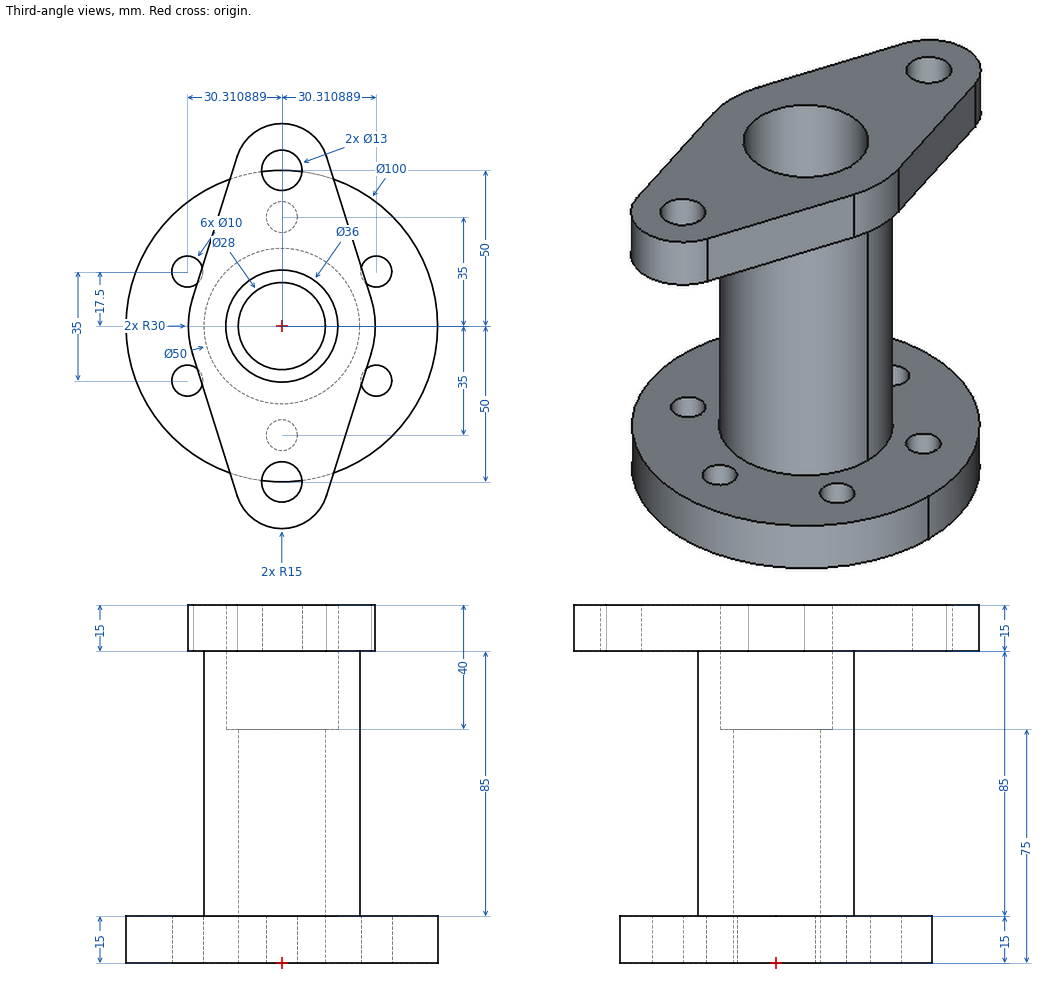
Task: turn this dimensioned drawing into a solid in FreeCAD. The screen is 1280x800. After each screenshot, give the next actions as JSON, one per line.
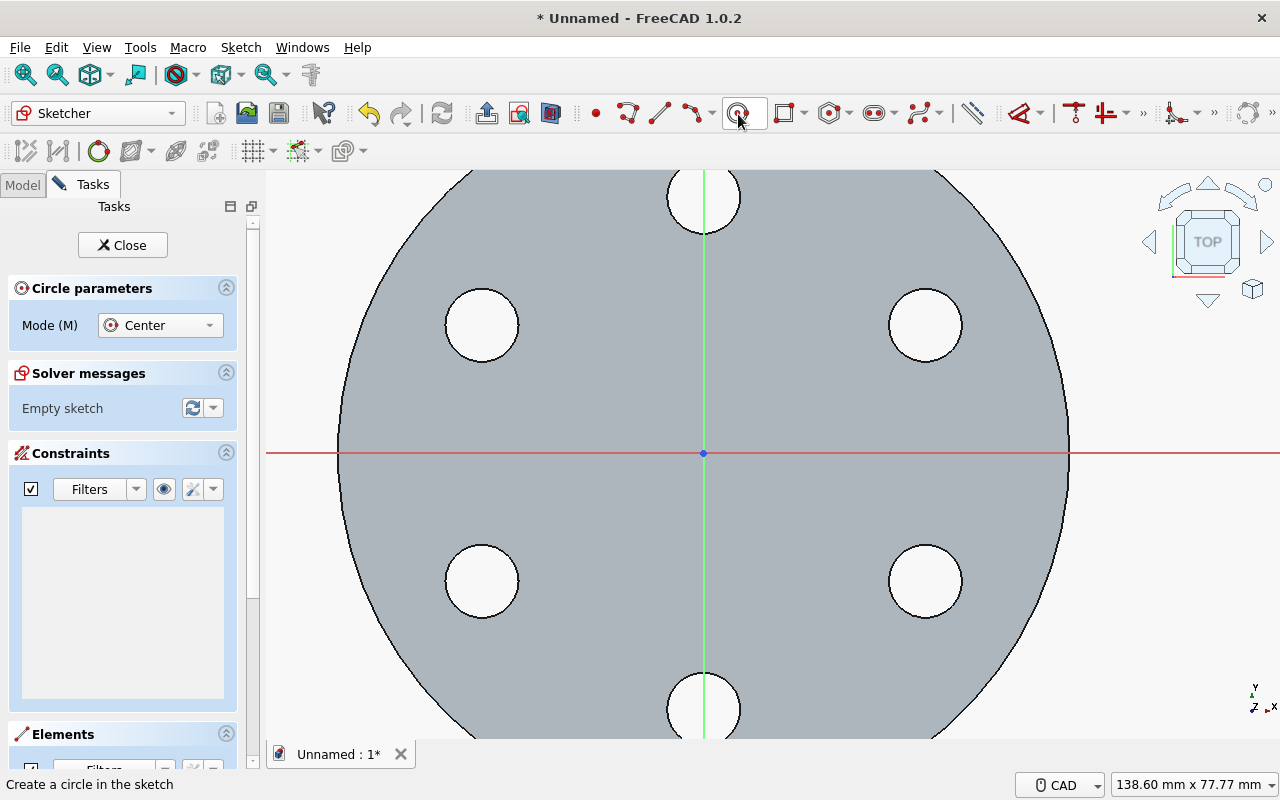
{"action": "left_click", "coordinate": [704, 453]}
{"action": "mouse_move", "coordinate": [833, 324]}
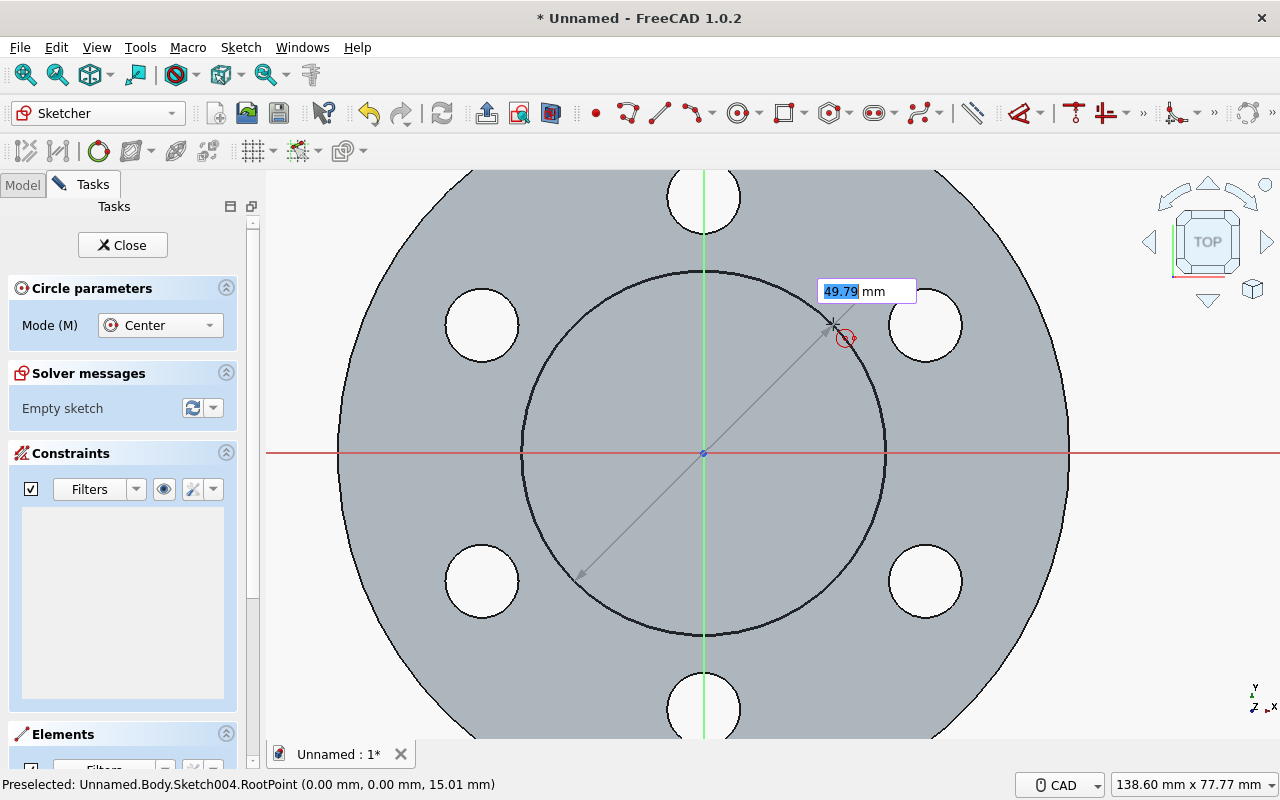
{"action": "type", "text": "50"}
{"action": "key", "text": "Return"}
{"action": "key", "text": "Escape"}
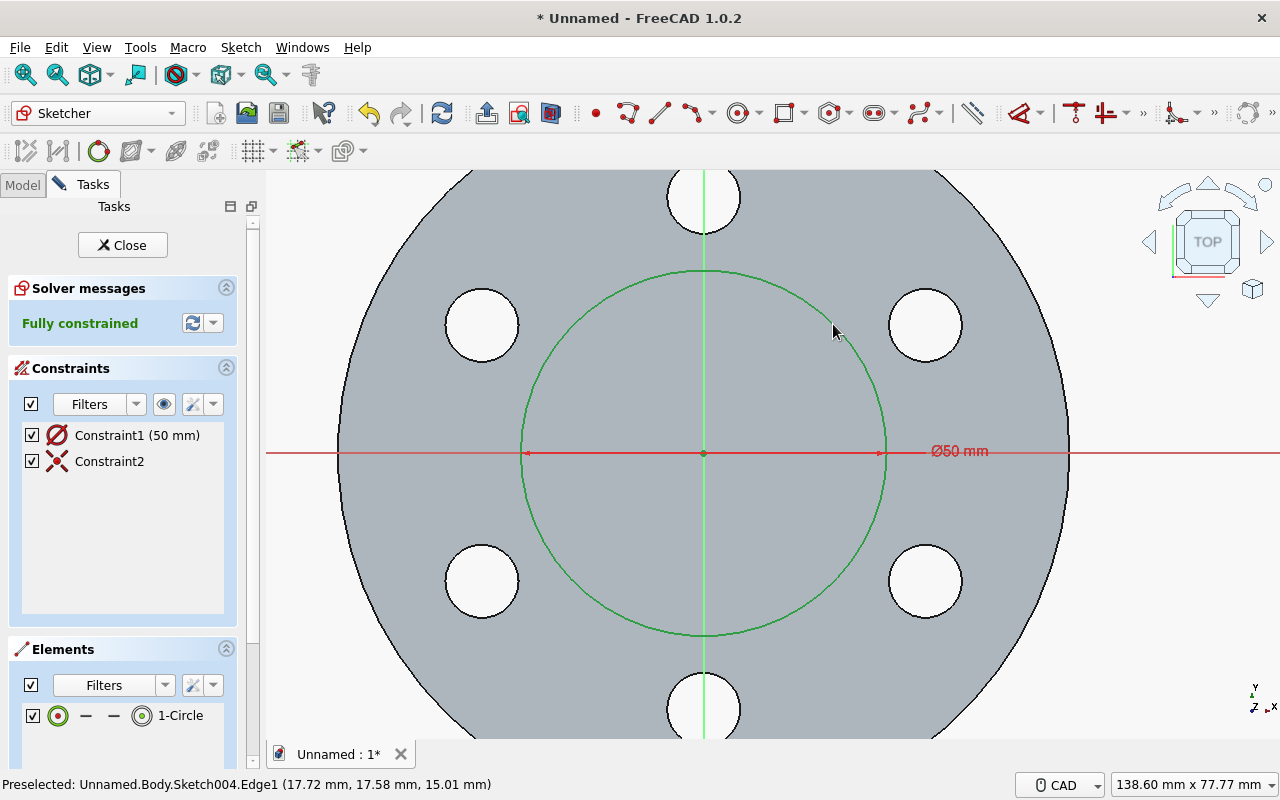
{"action": "left_click", "coordinate": [123, 245]}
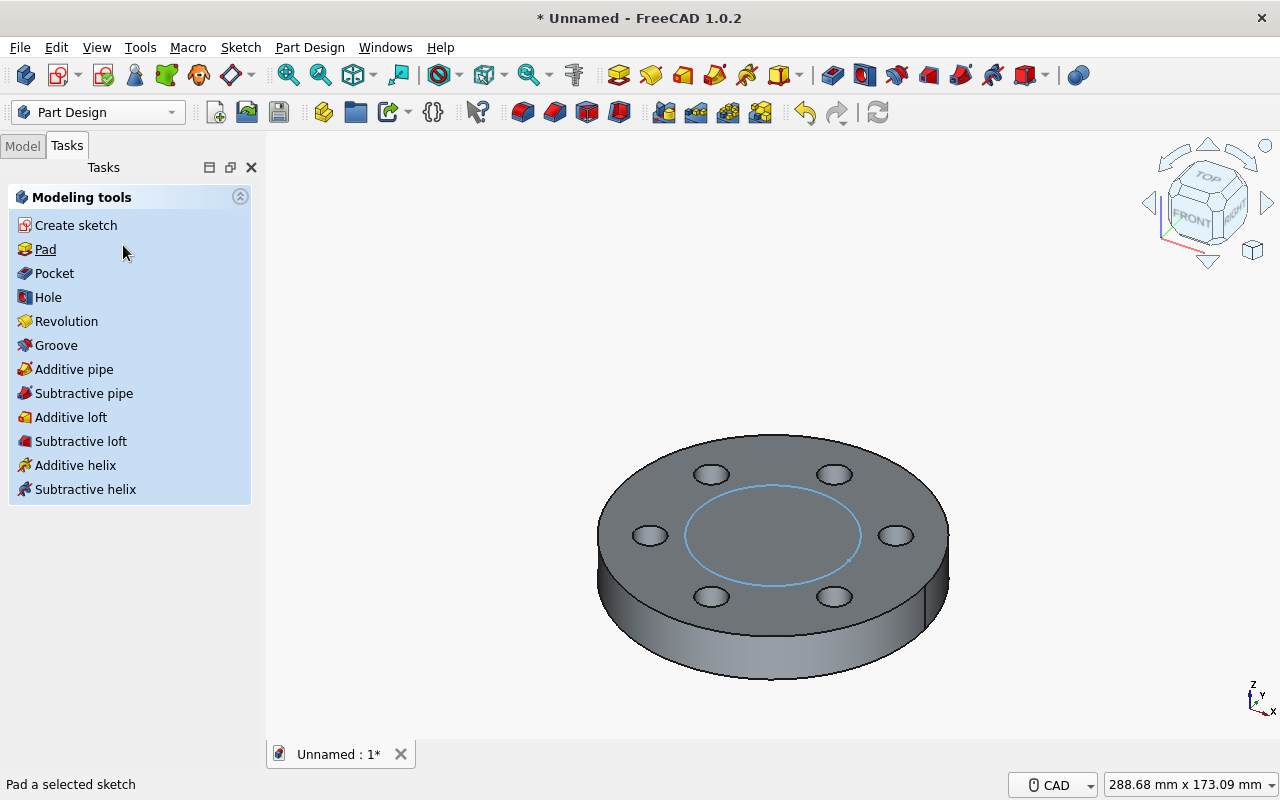
{"action": "left_click", "coordinate": [620, 76]}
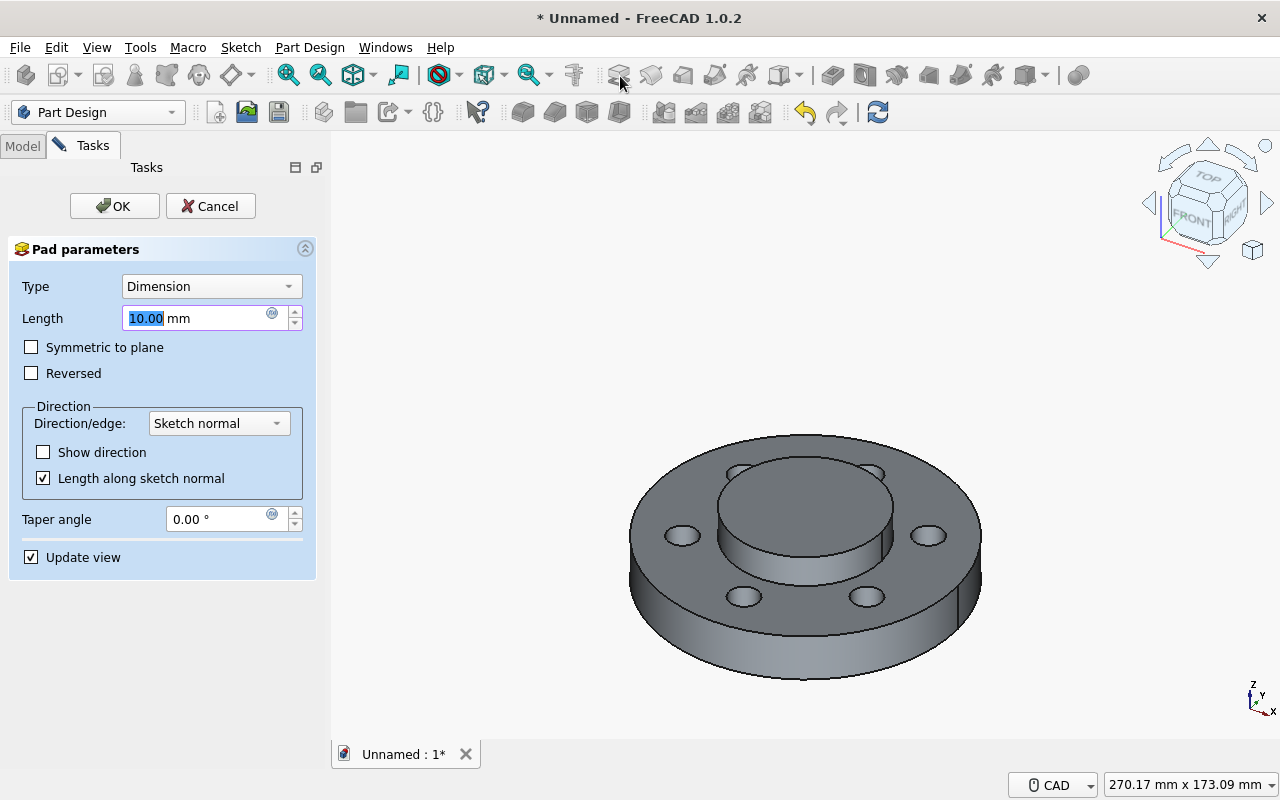
{"action": "type", "text": "85"}
{"action": "key", "text": "Tab"}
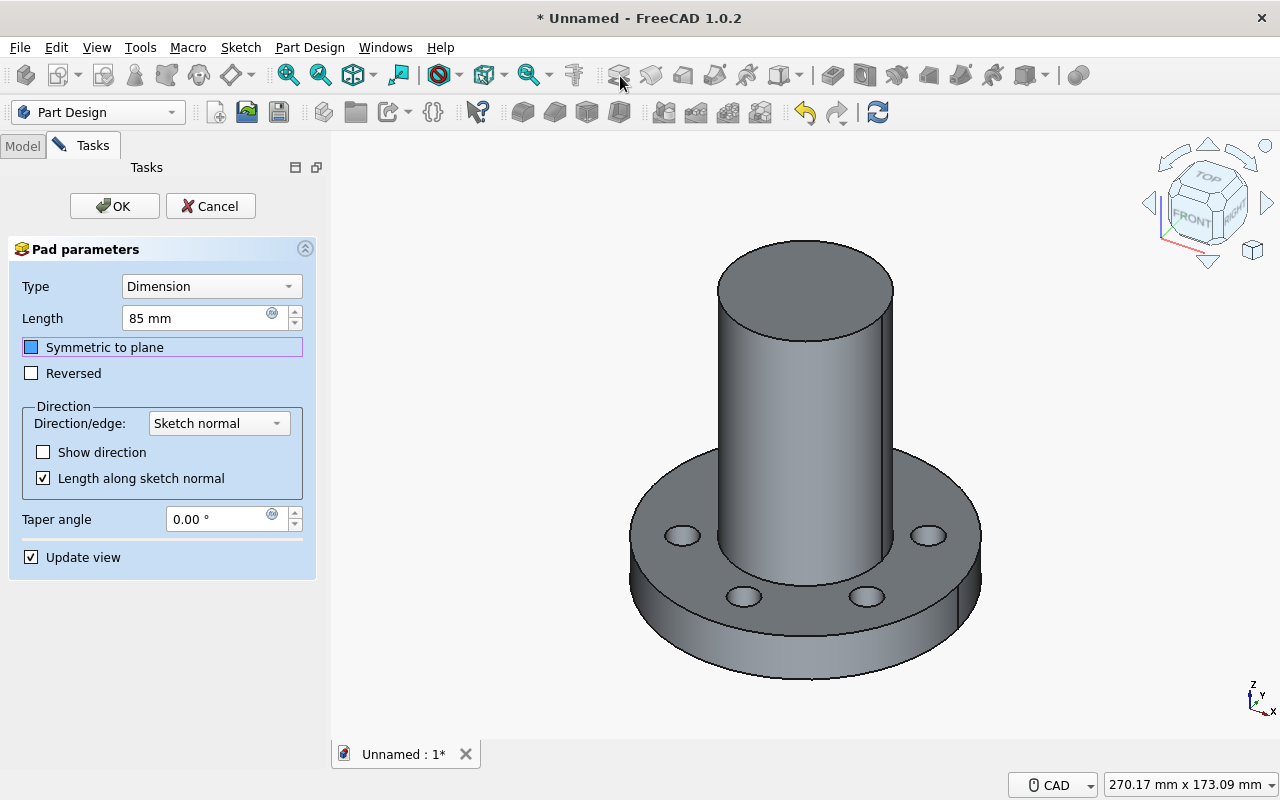
{"action": "left_click", "coordinate": [115, 206]}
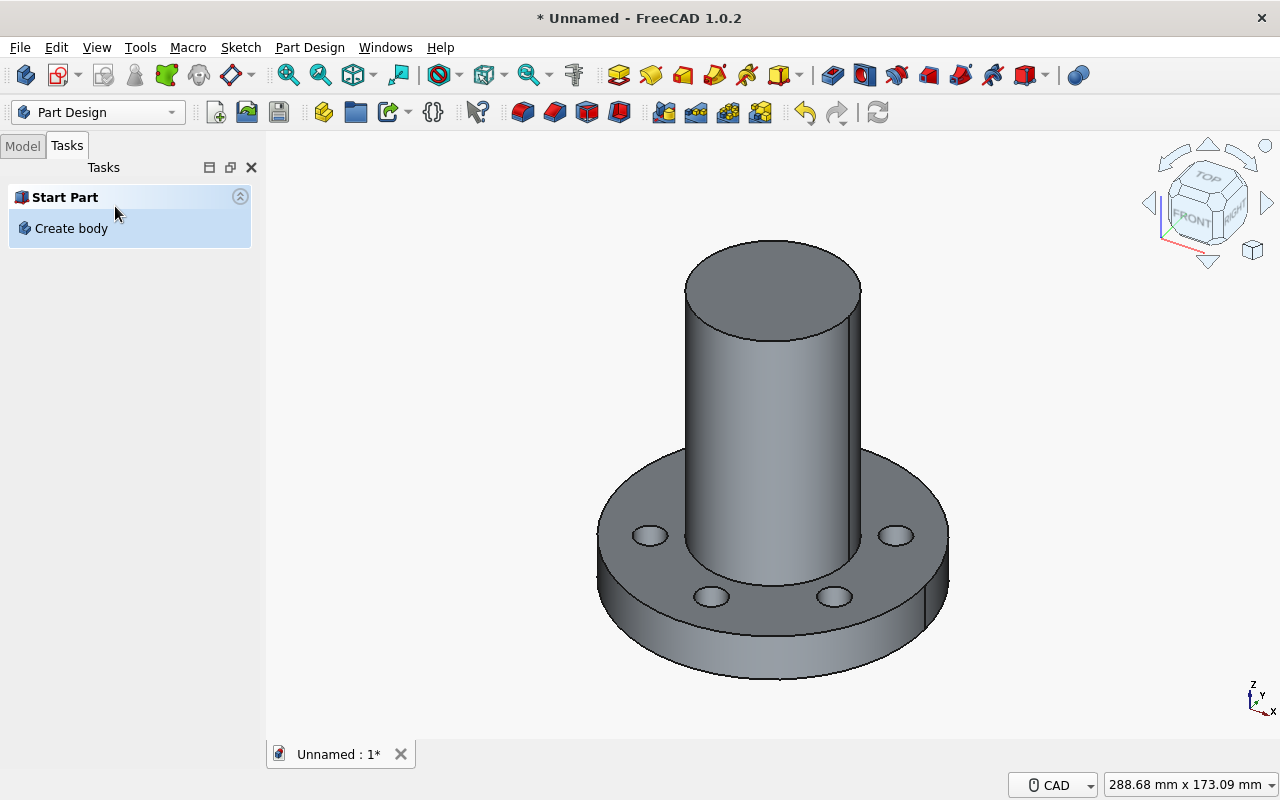
{"action": "left_click", "coordinate": [773, 290]}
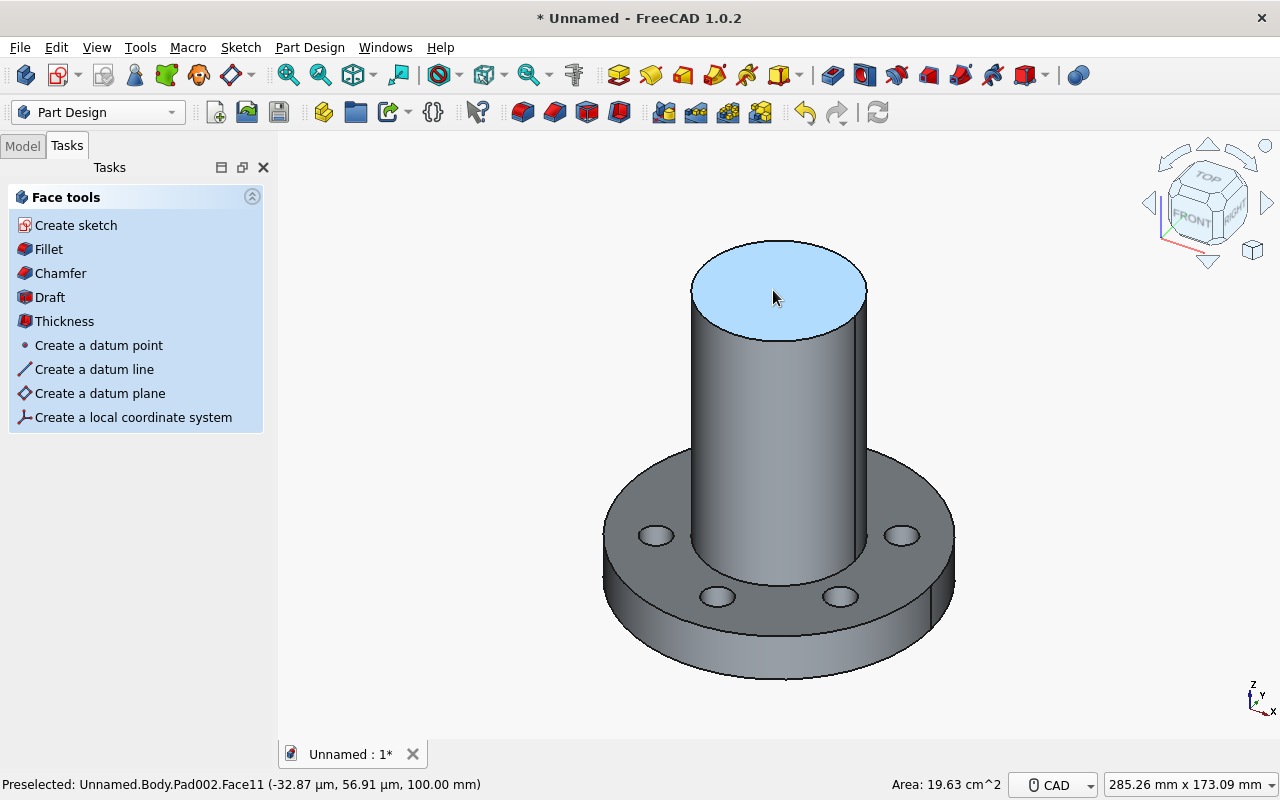
{"action": "left_click", "coordinate": [58, 76]}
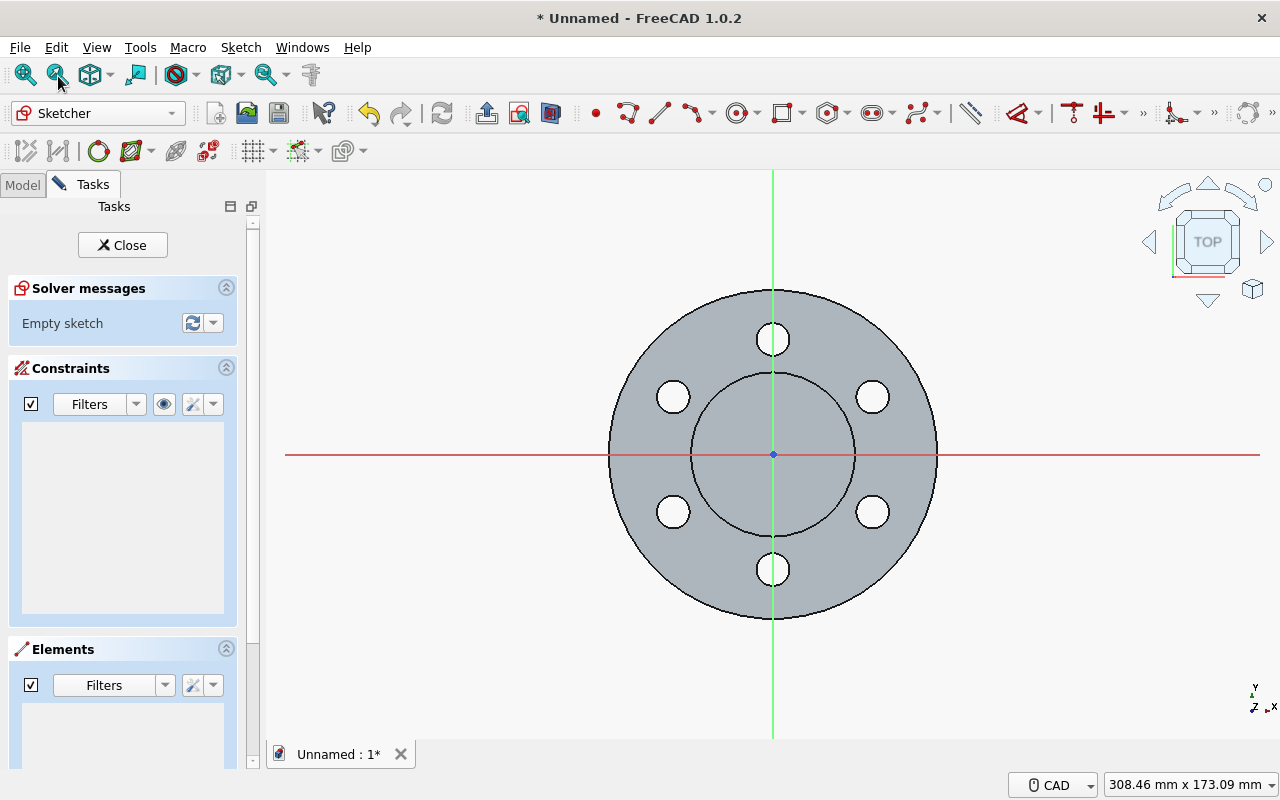
{"action": "key", "text": "g l"}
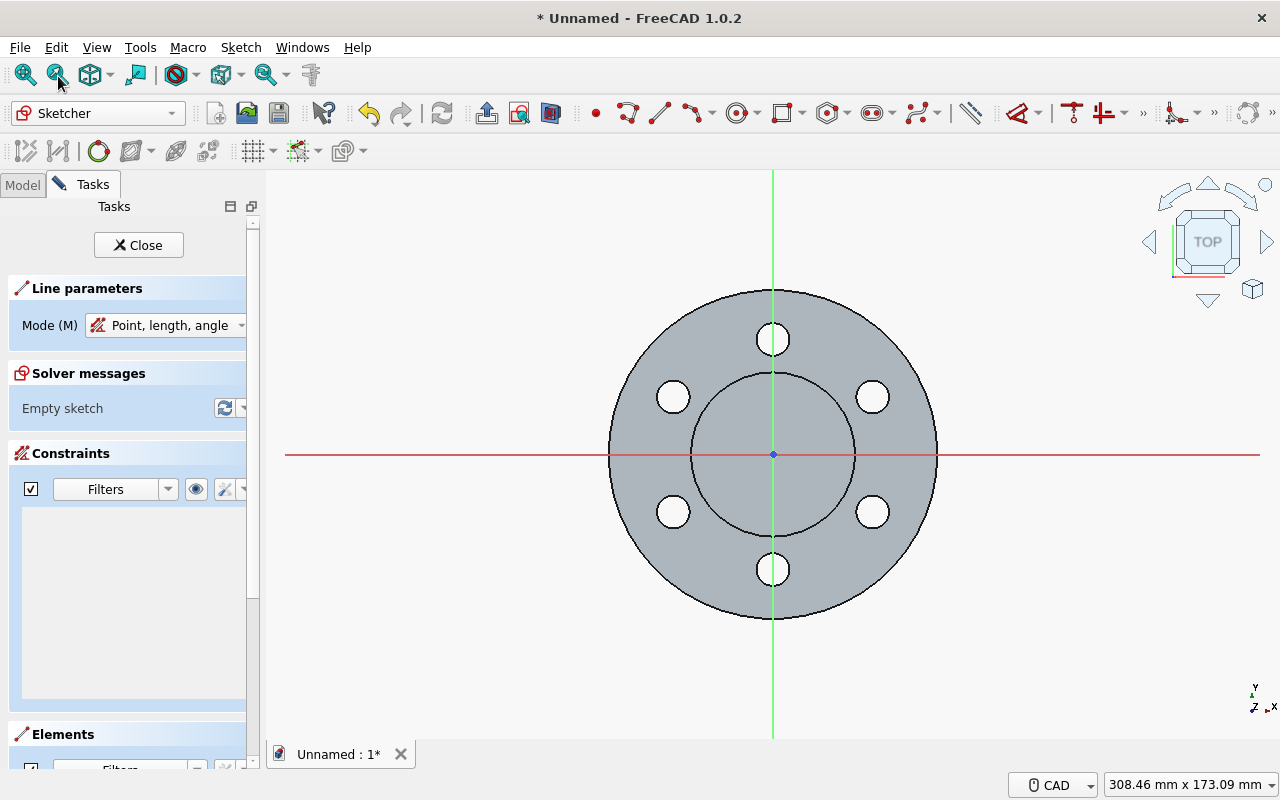
{"action": "left_click", "coordinate": [726, 275]}
{"action": "left_click", "coordinate": [679, 425]}